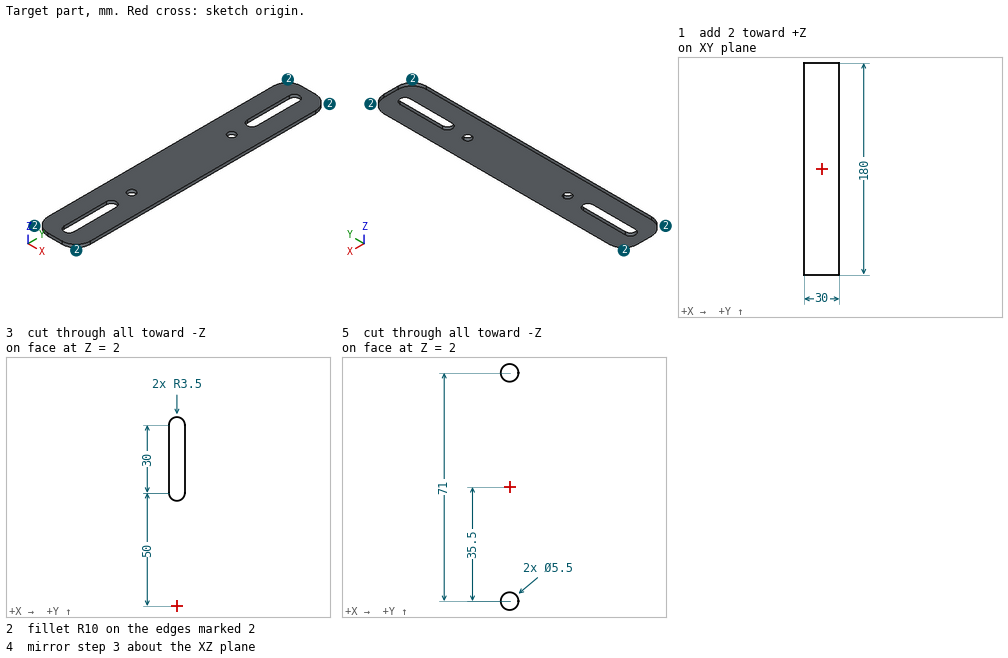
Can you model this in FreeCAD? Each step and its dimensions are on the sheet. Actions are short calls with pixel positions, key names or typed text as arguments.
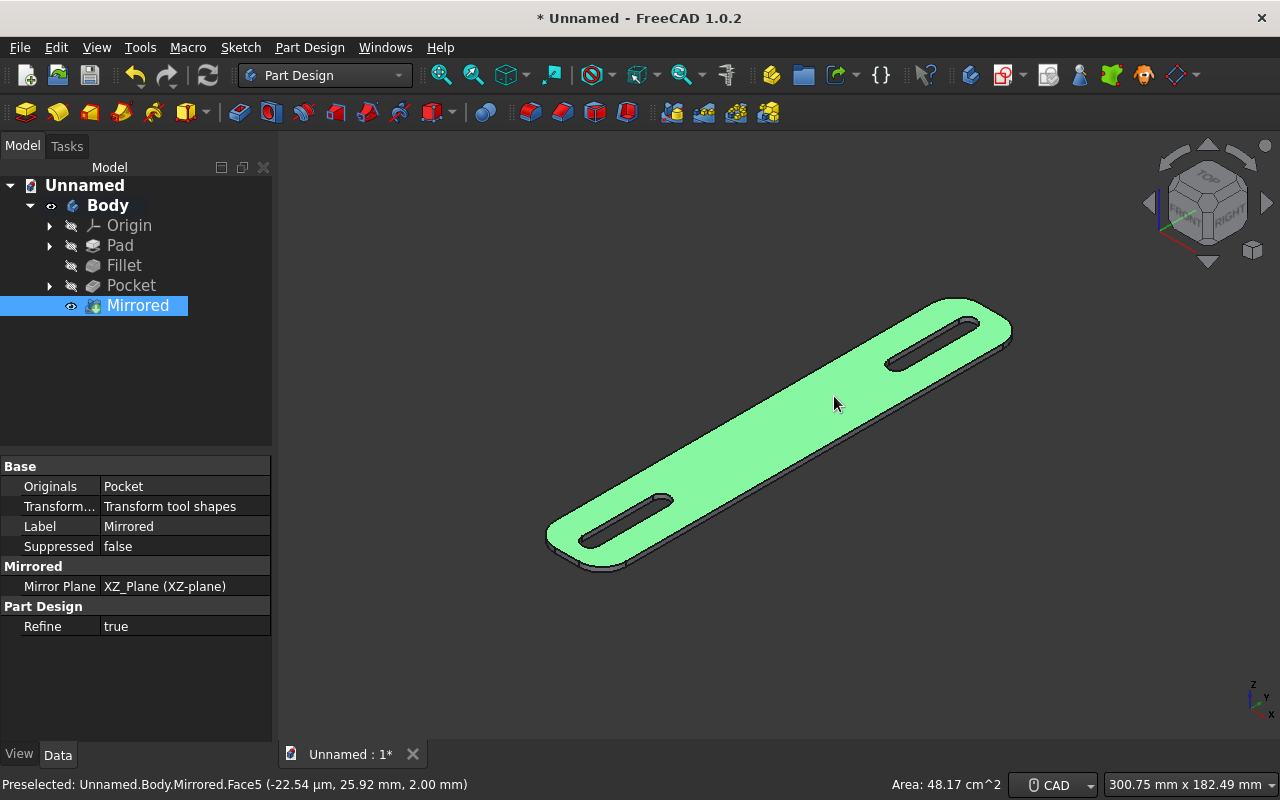
click(1004, 76)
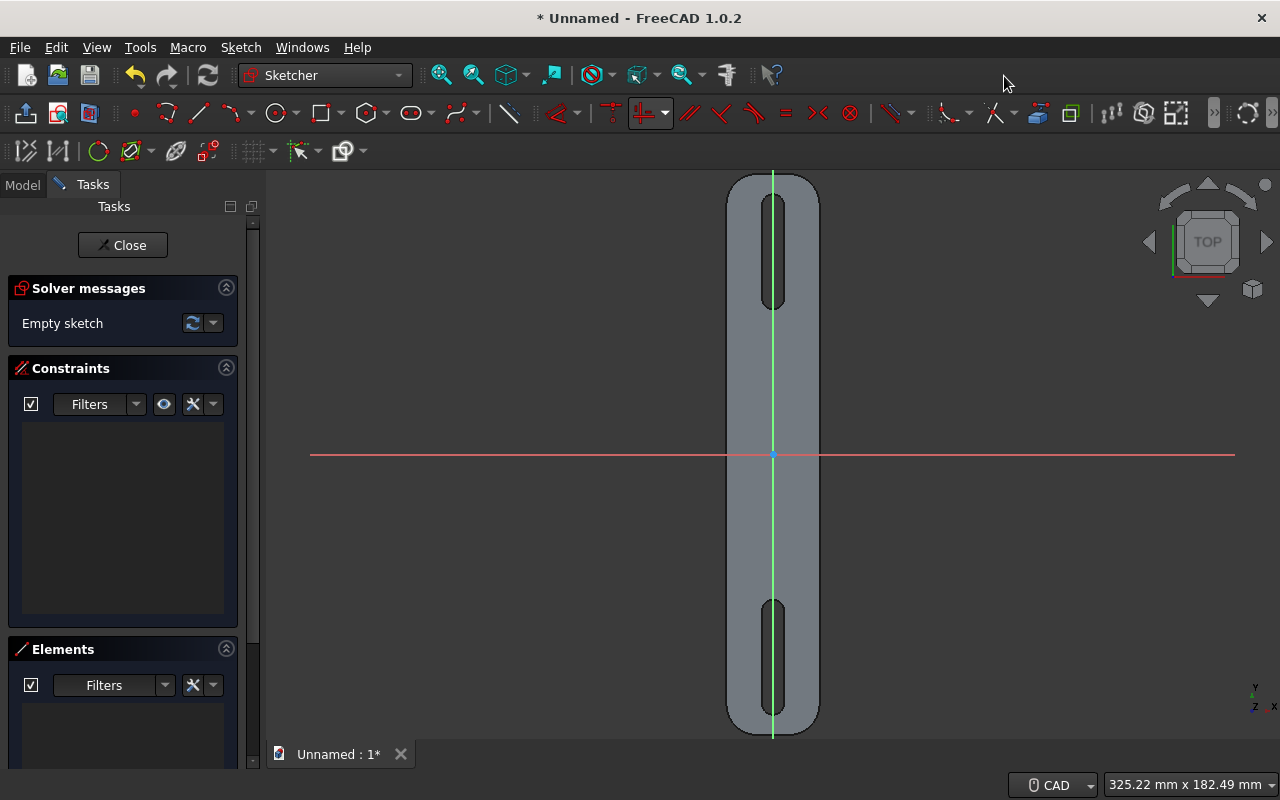
scroll(912, 454, up, 2)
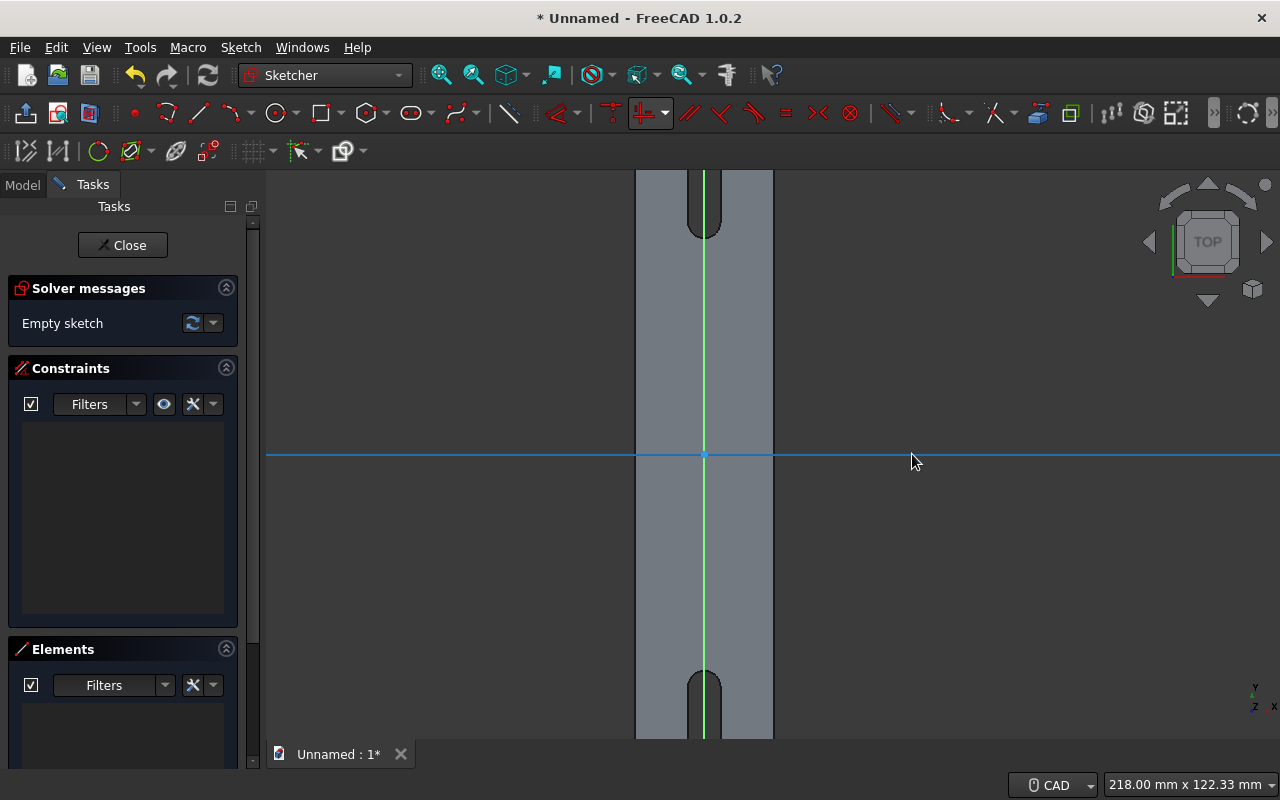
click(276, 114)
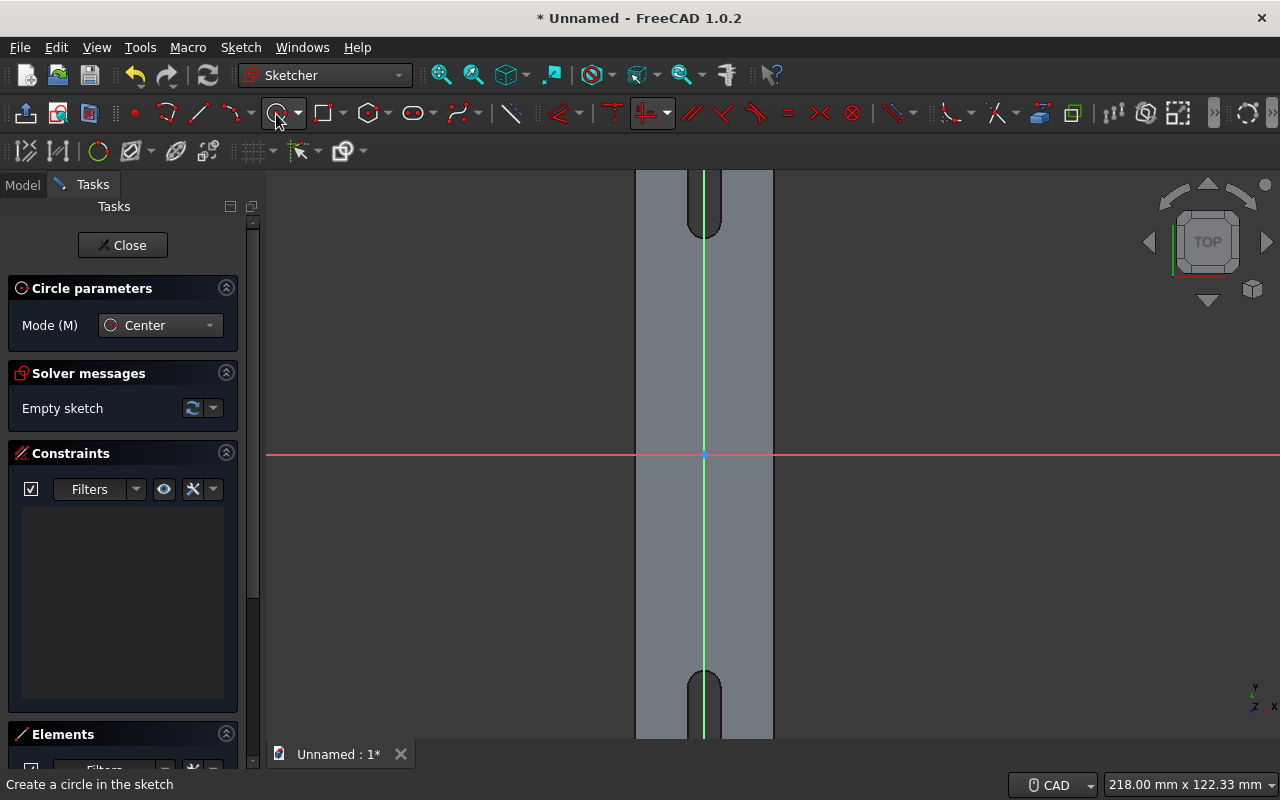
scroll(704, 620, up, 3)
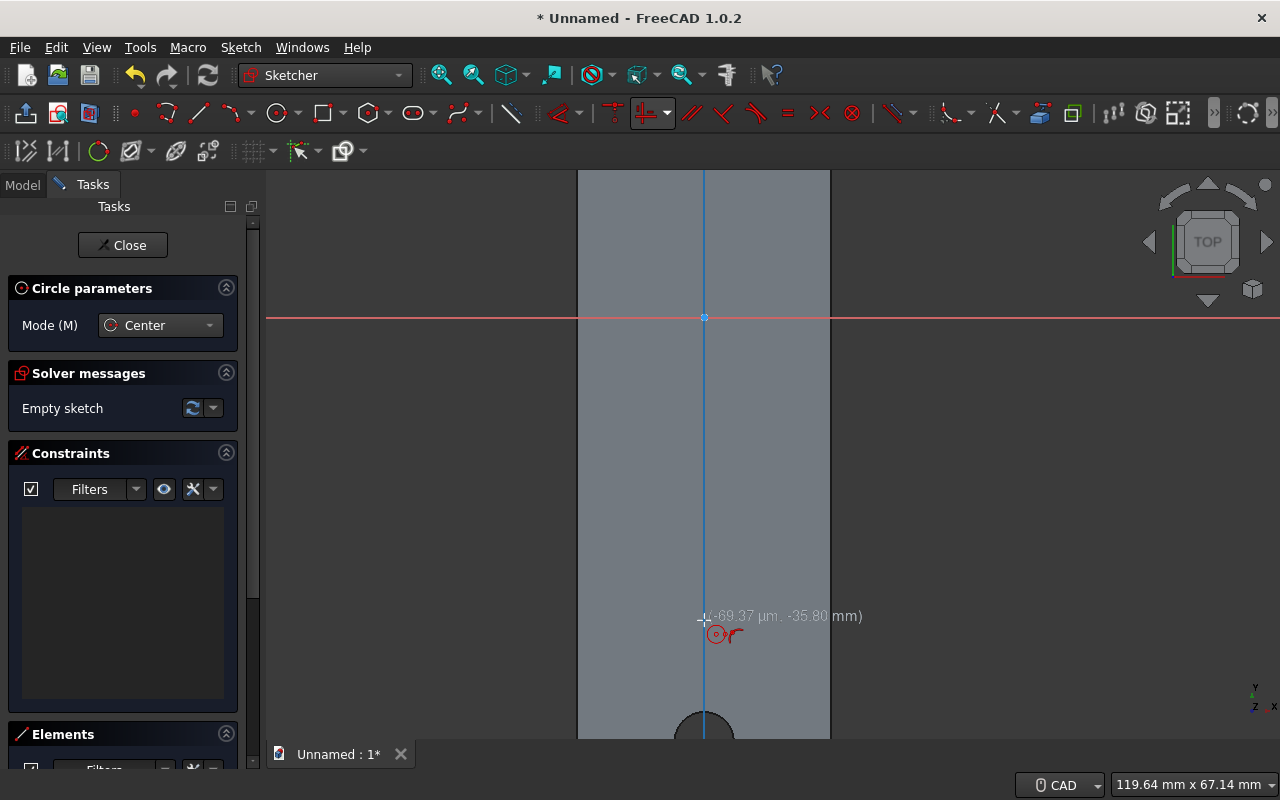
click(704, 619)
click(721, 602)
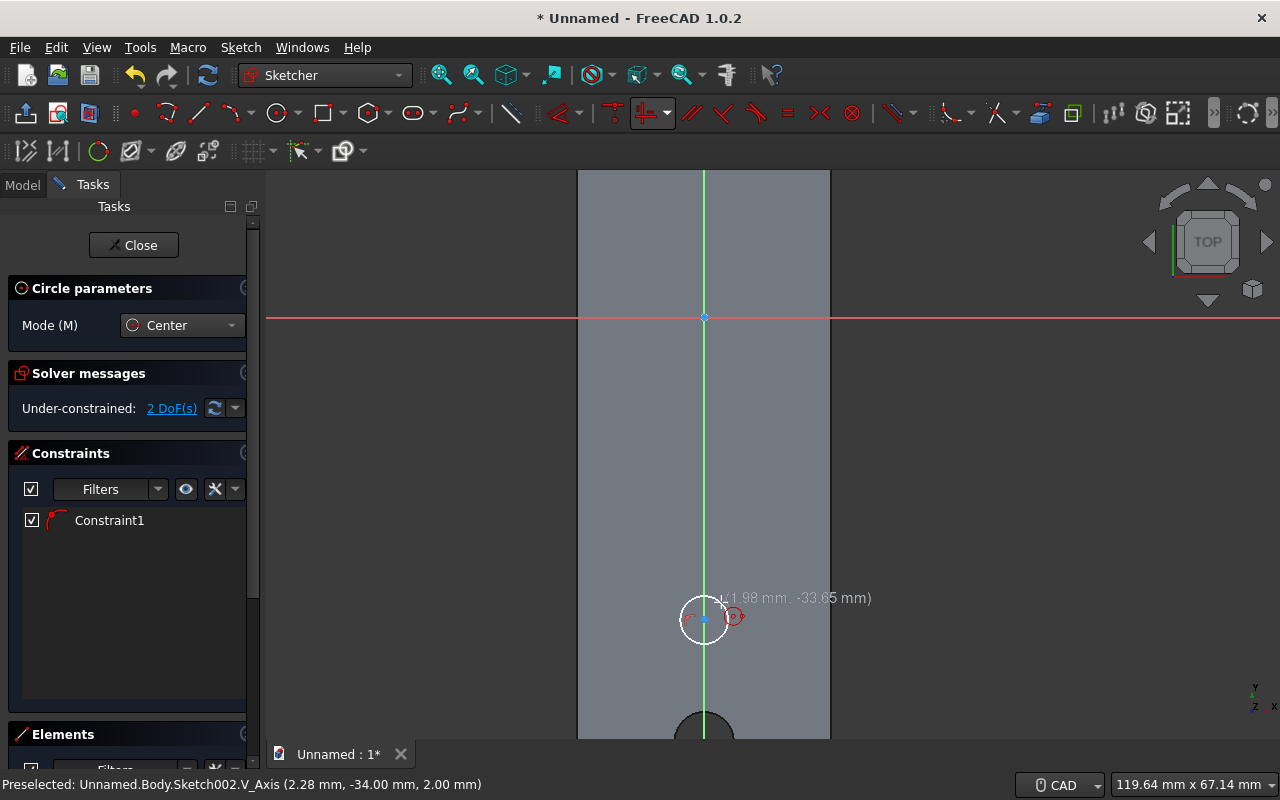
scroll(705, 621, down, 3)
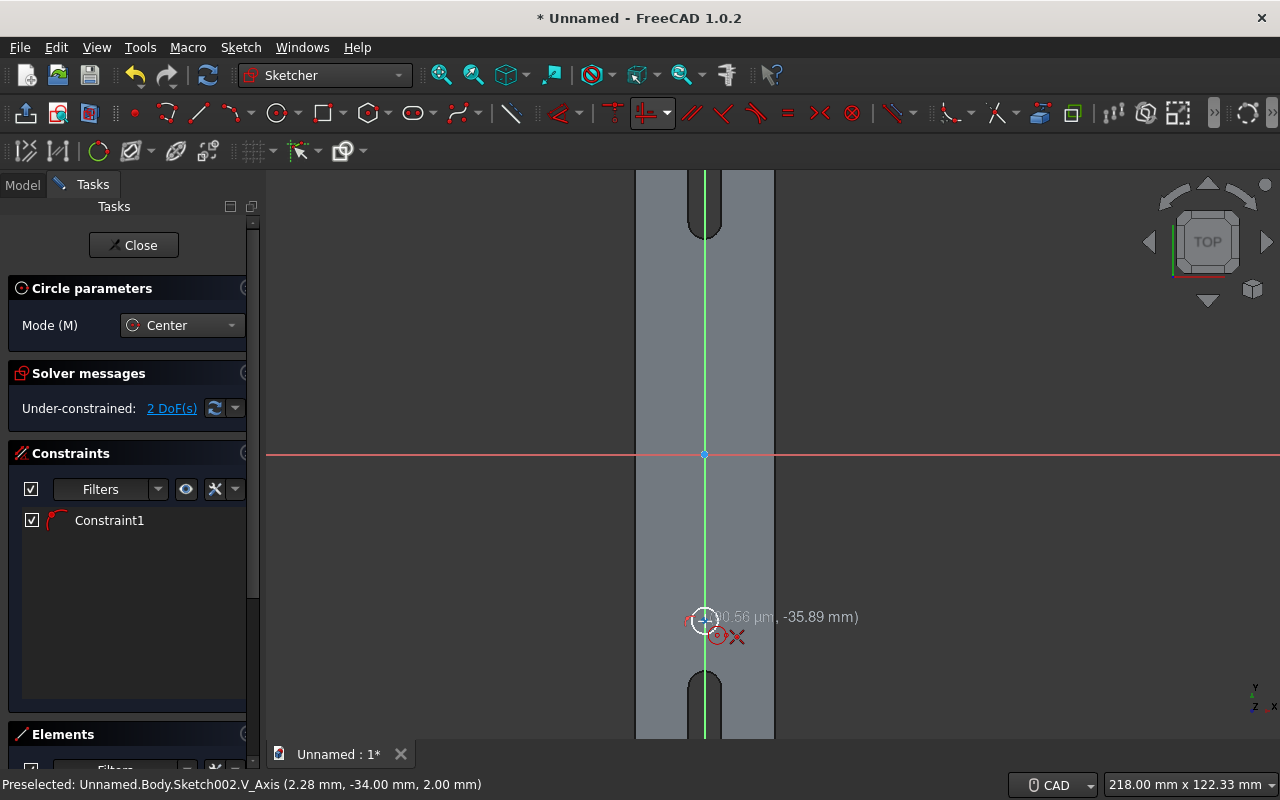
scroll(705, 290, up, 3)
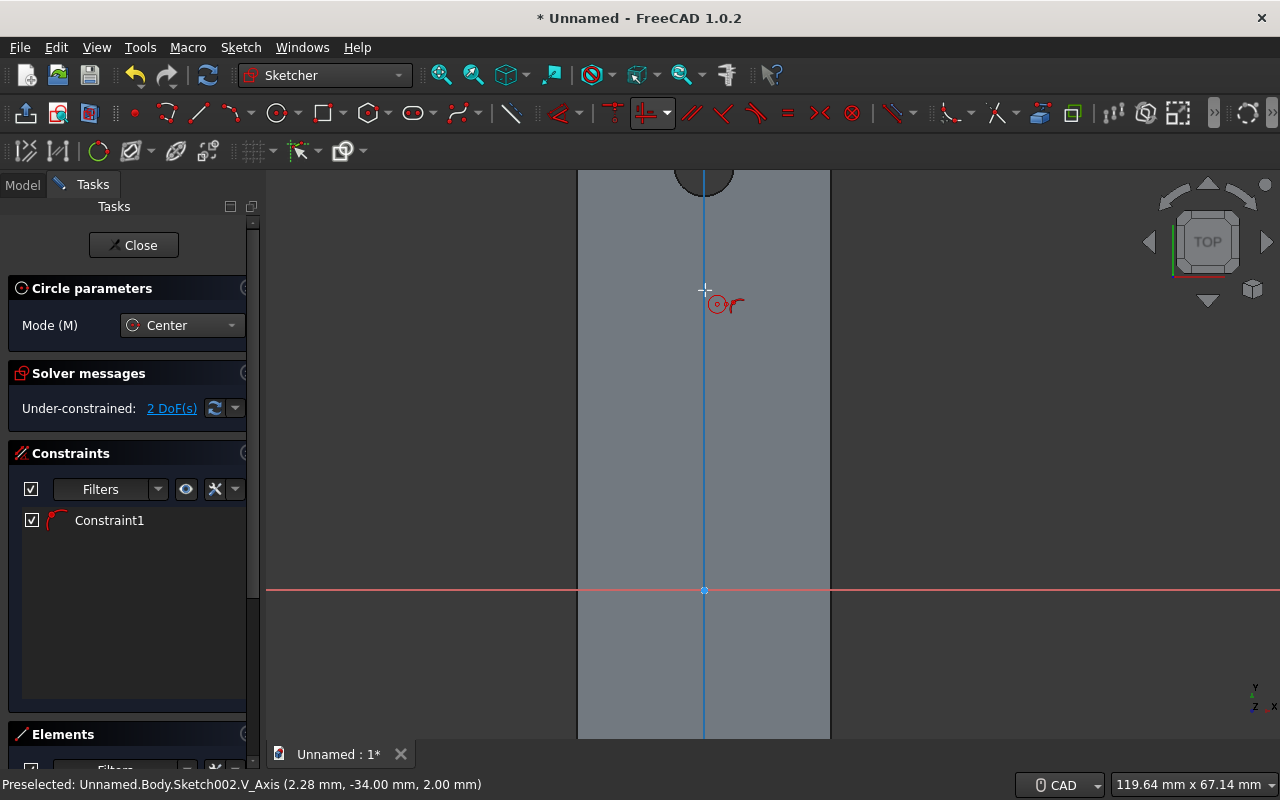
click(704, 290)
click(721, 273)
key(Escape)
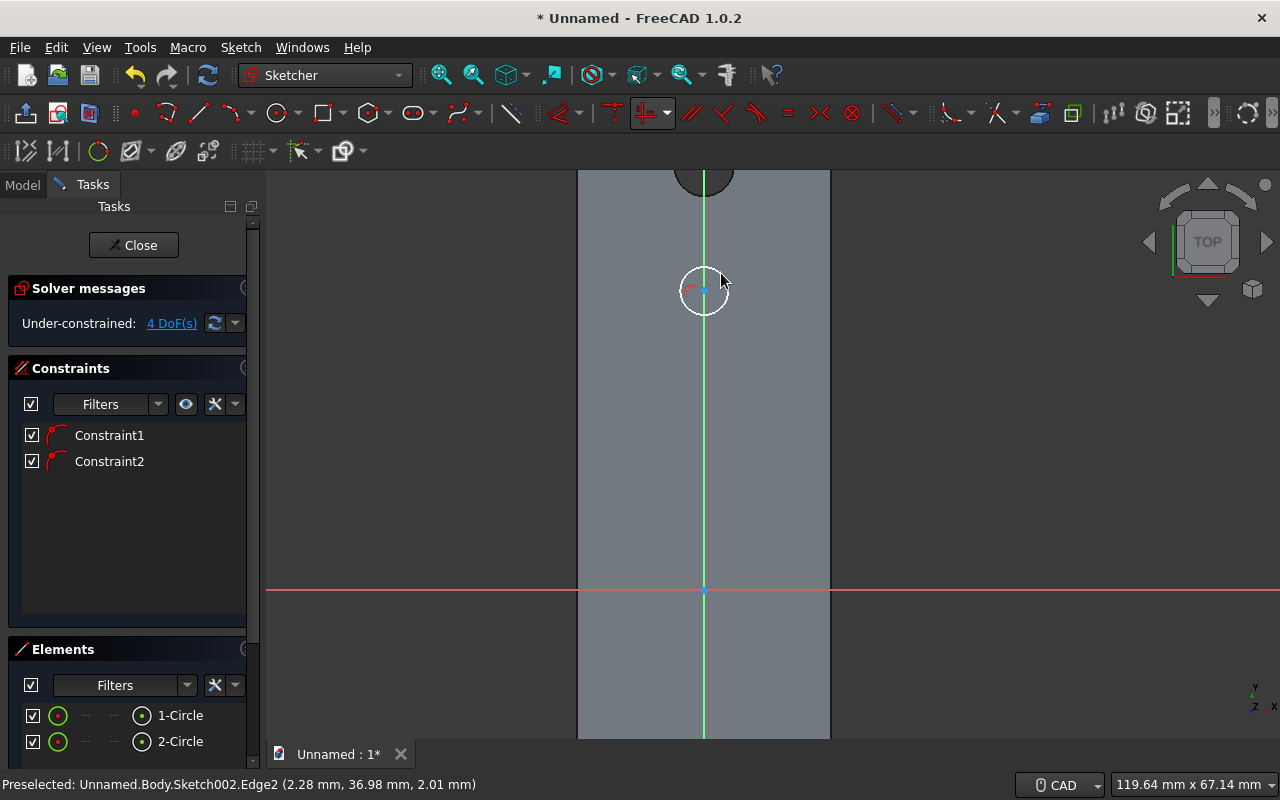
scroll(705, 289, down, 3)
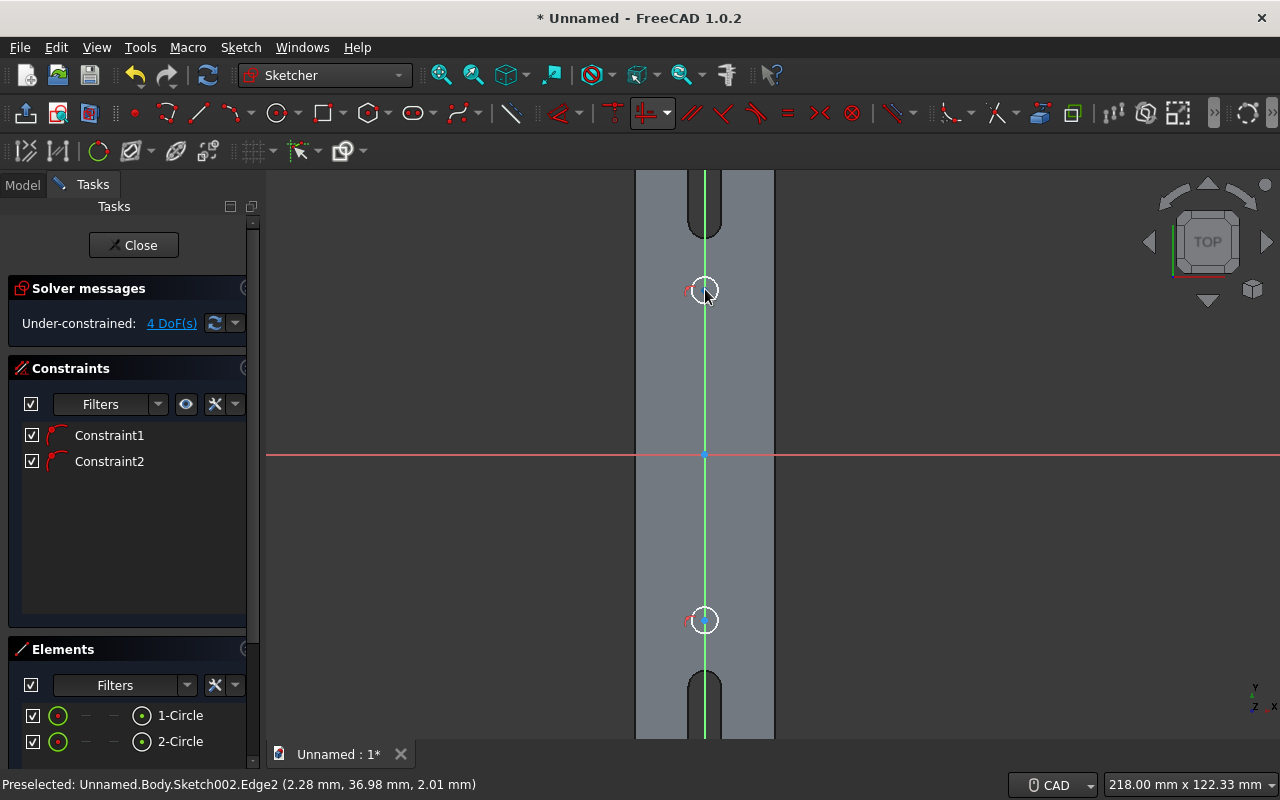
scroll(714, 611, up, 3)